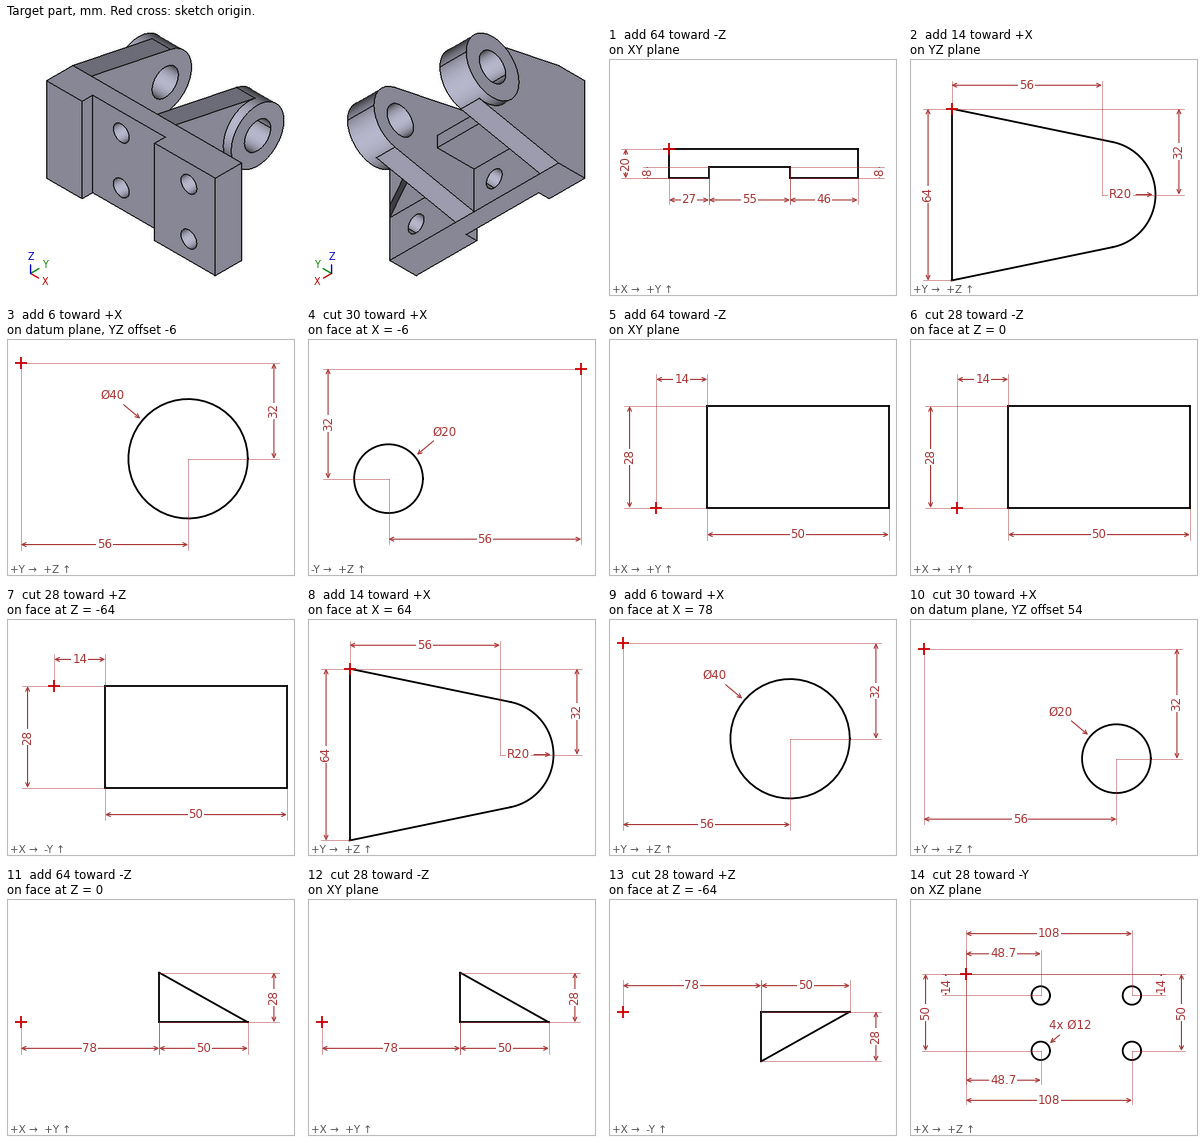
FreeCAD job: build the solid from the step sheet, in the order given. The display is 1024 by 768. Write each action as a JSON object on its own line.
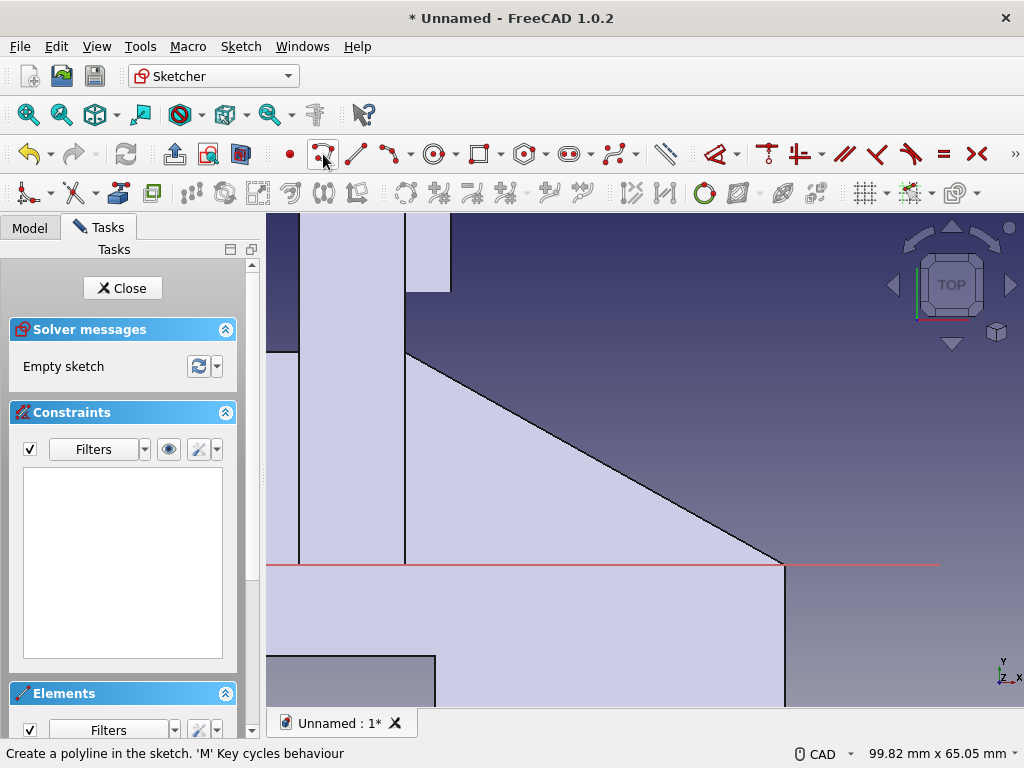
{"action": "left_click", "coordinate": [405, 565]}
{"action": "left_click", "coordinate": [785, 556]}
{"action": "left_click", "coordinate": [405, 352]}
{"action": "left_click", "coordinate": [405, 565]}
{"action": "key", "text": "Escape"}
{"action": "key", "text": "Escape"}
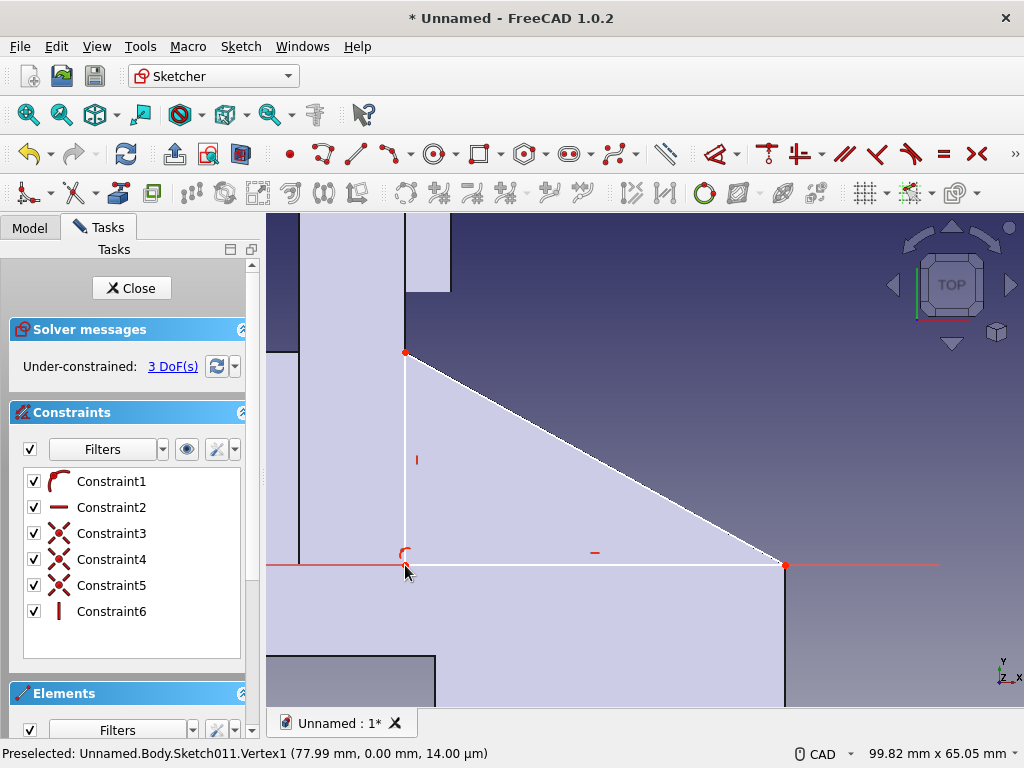
{"action": "left_click", "coordinate": [714, 154]}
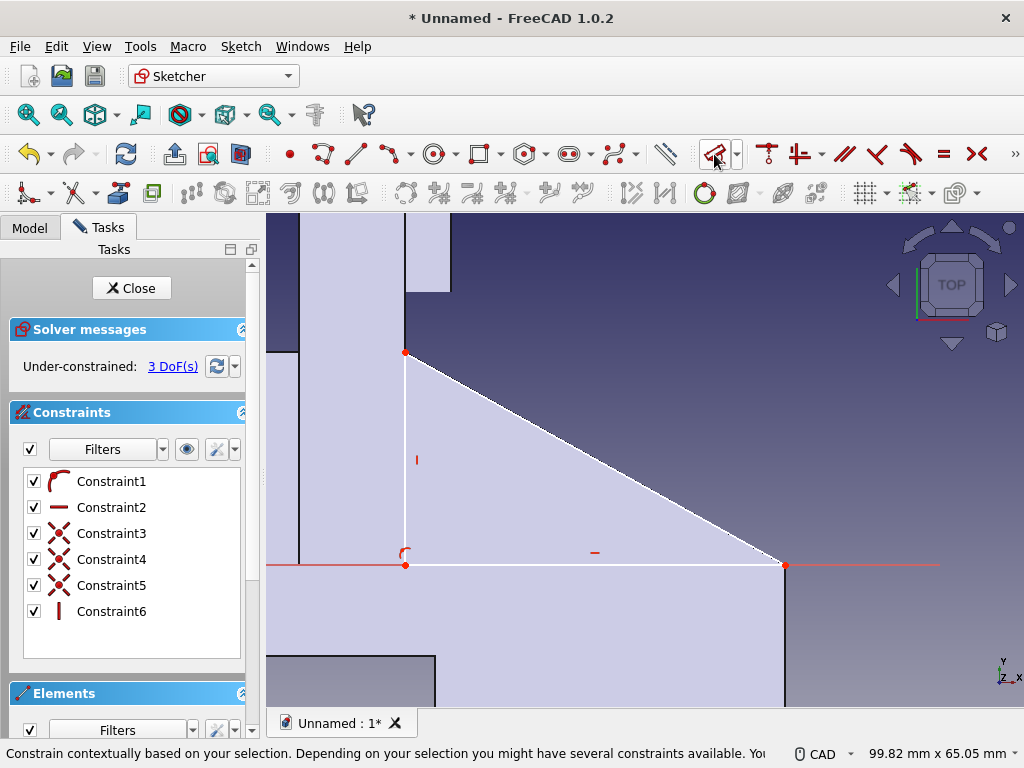
{"action": "left_click", "coordinate": [519, 565]}
{"action": "left_click", "coordinate": [595, 599]}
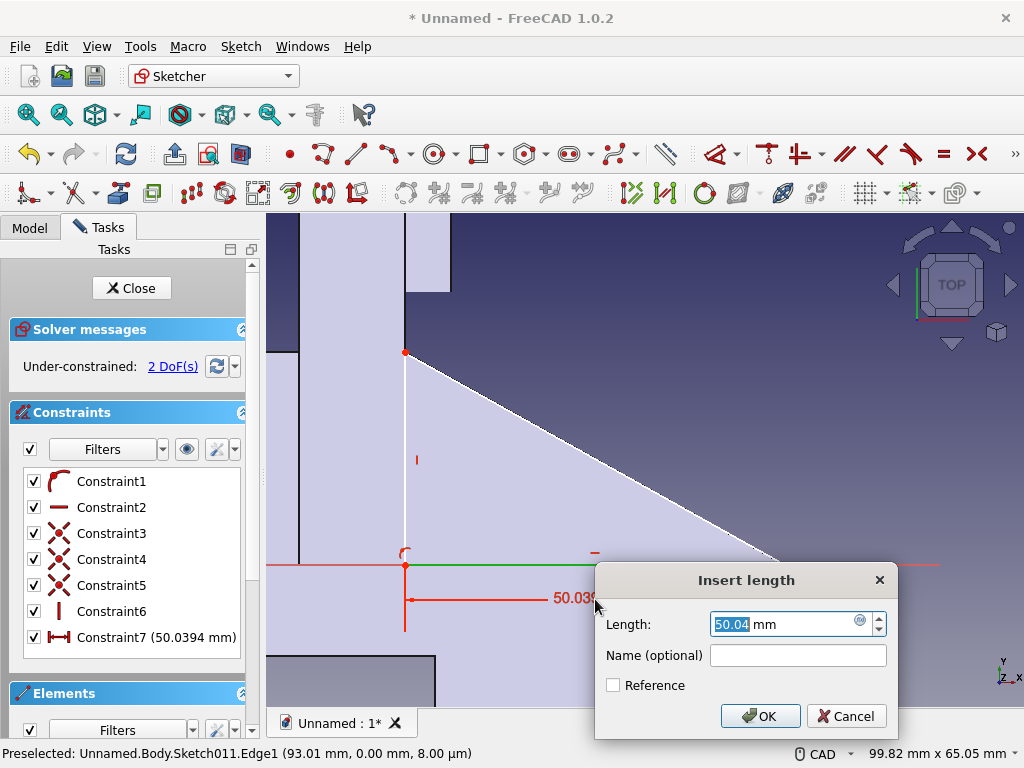
{"action": "type", "text": "50"}
{"action": "key", "text": "Return"}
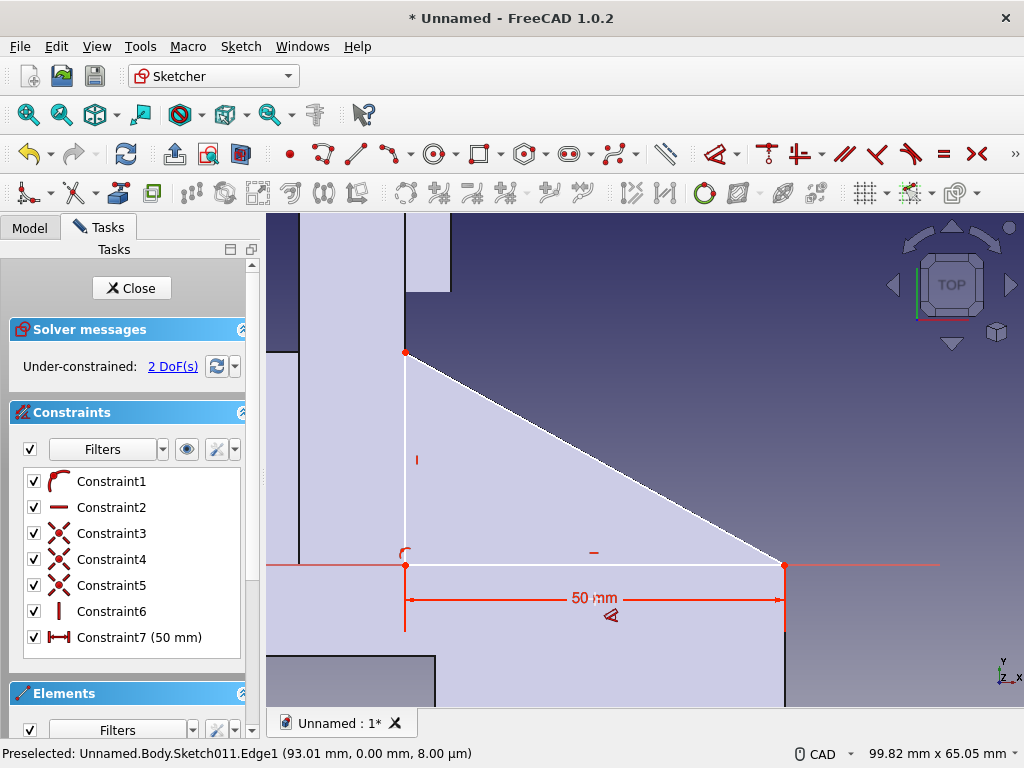
{"action": "left_click", "coordinate": [405, 417]}
{"action": "left_click", "coordinate": [371, 459]}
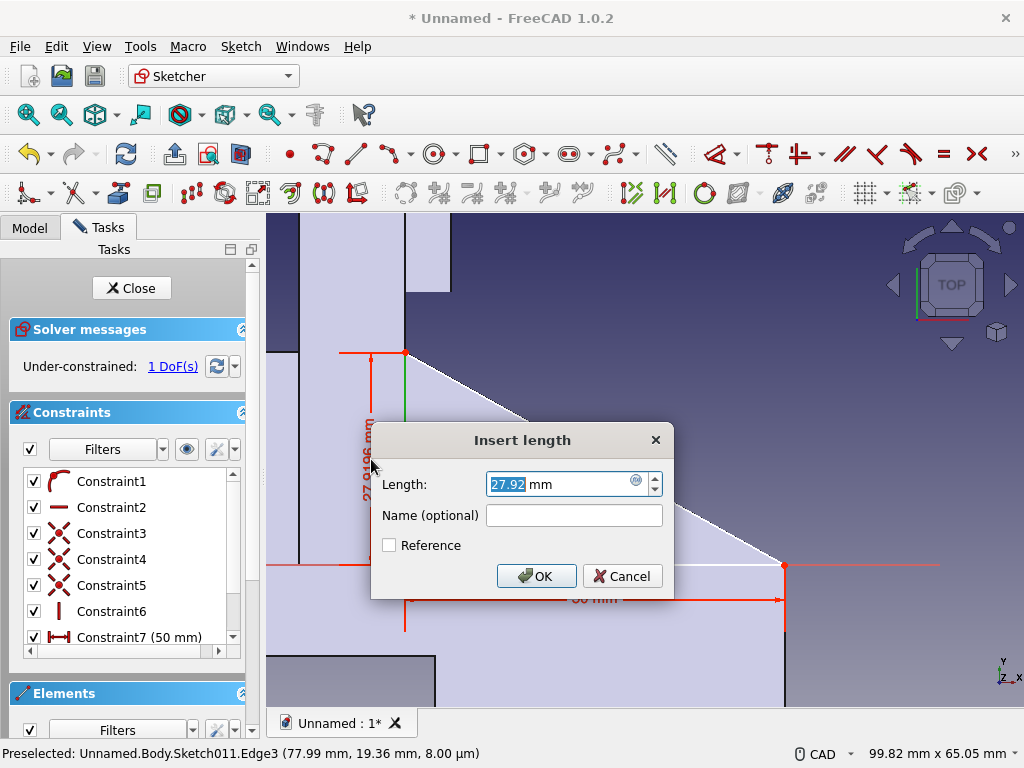
{"action": "type", "text": "28"}
{"action": "key", "text": "Return"}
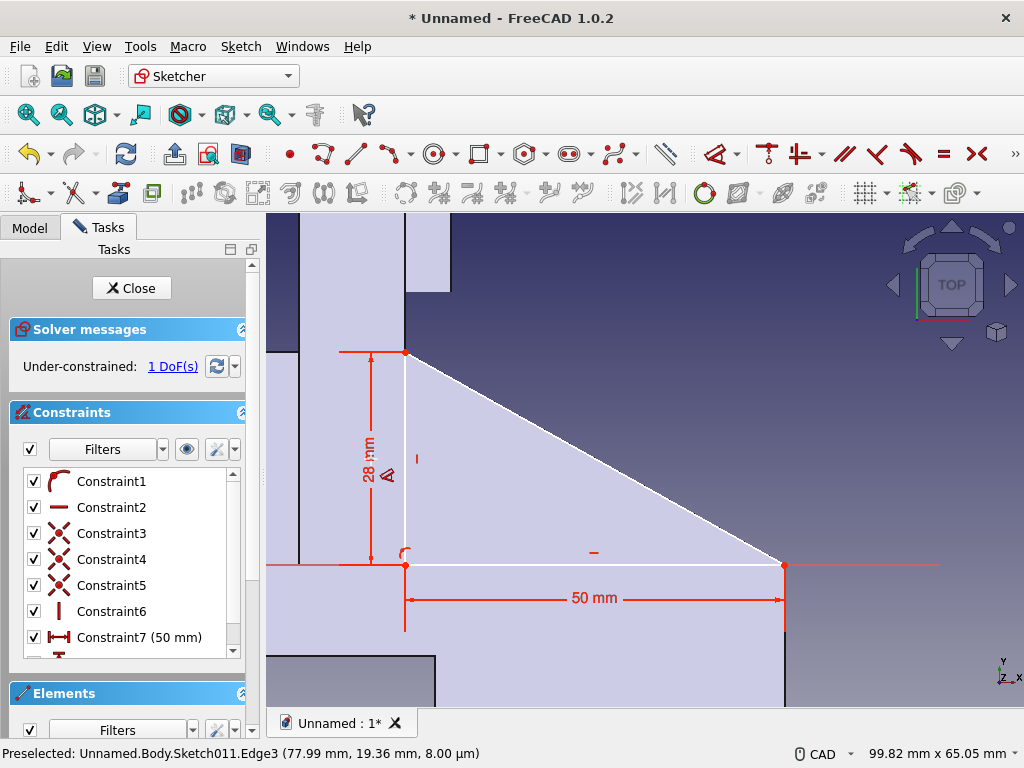
{"action": "left_click", "coordinate": [405, 565]}
{"action": "left_click", "coordinate": [350, 599]}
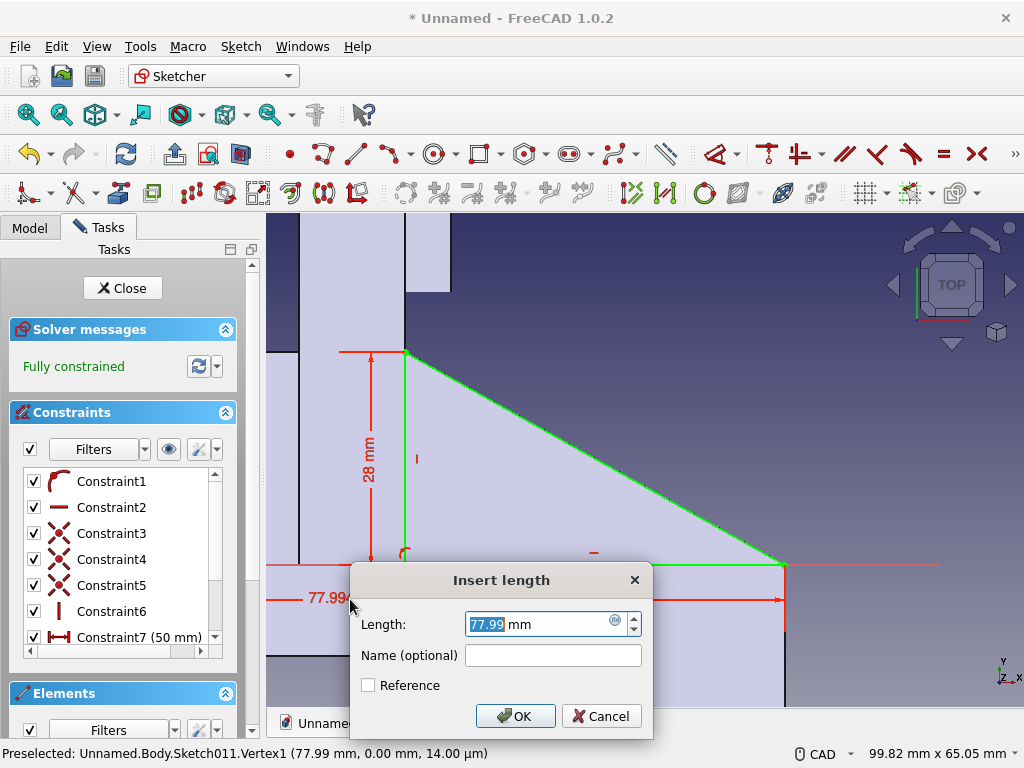
{"action": "type", "text": "78"}
{"action": "key", "text": "Return"}
{"action": "key", "text": "Escape"}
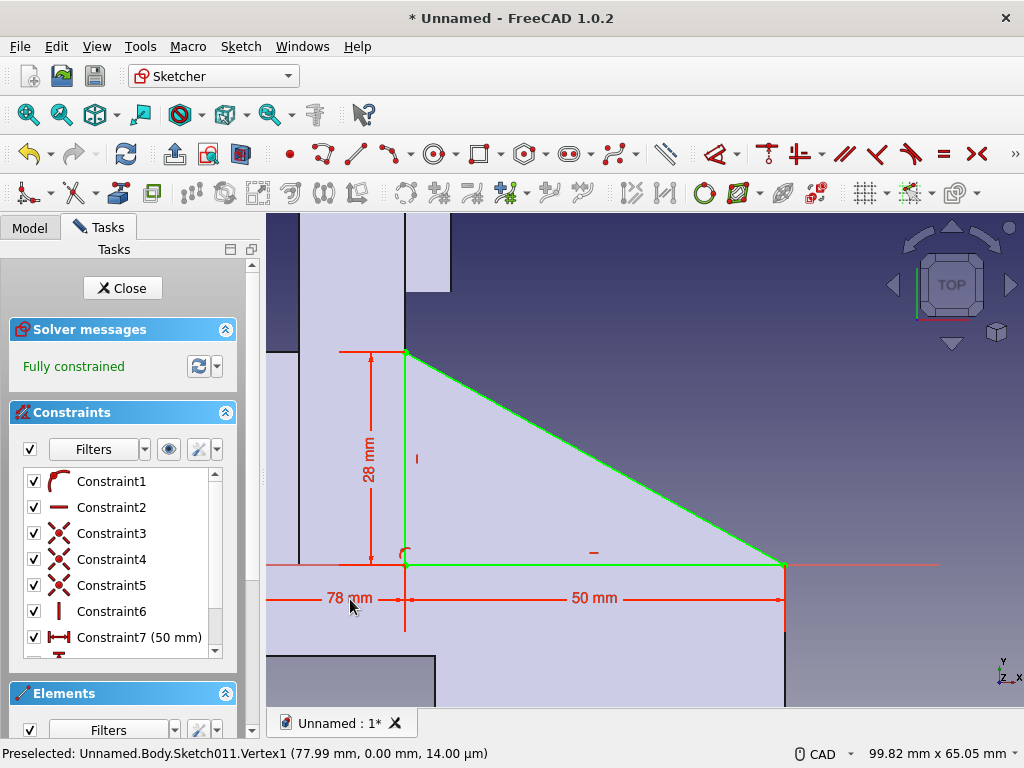
{"action": "left_click", "coordinate": [123, 288]}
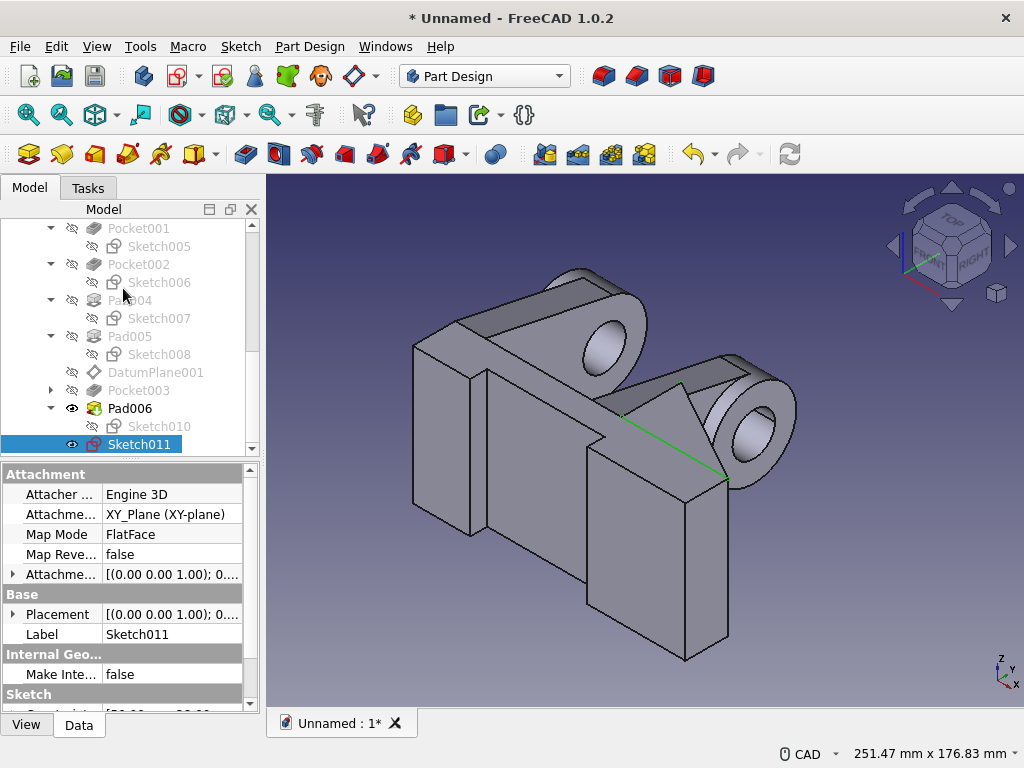
{"action": "left_click", "coordinate": [246, 154]}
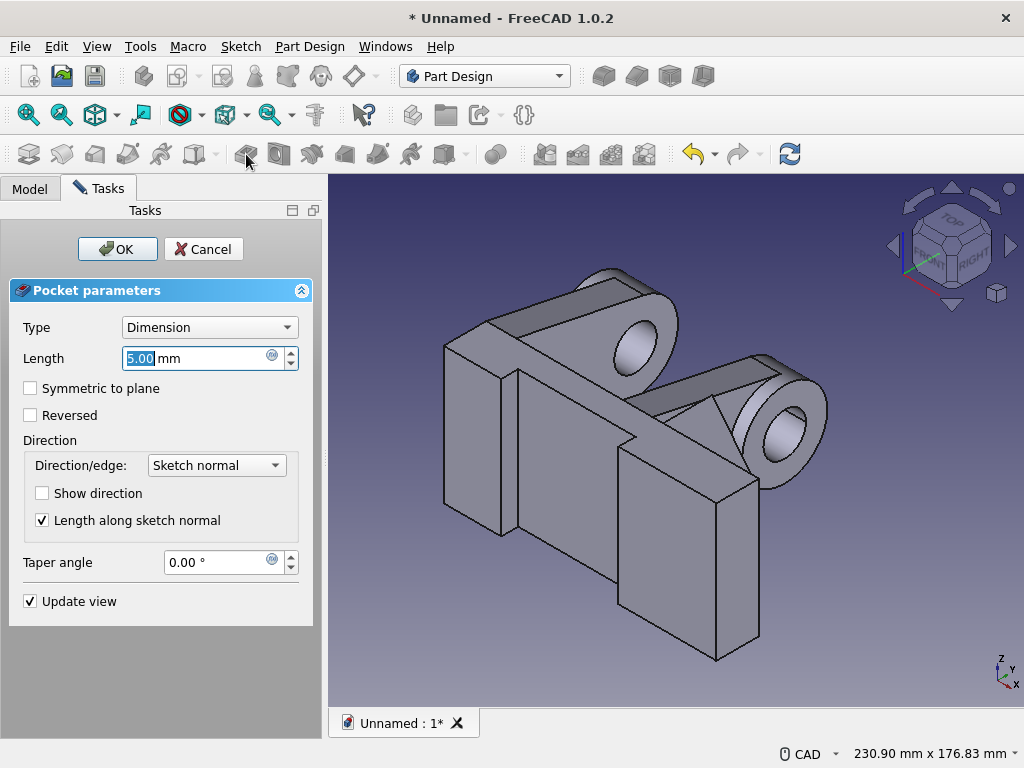
{"action": "type", "text": "28"}
{"action": "key", "text": "Tab"}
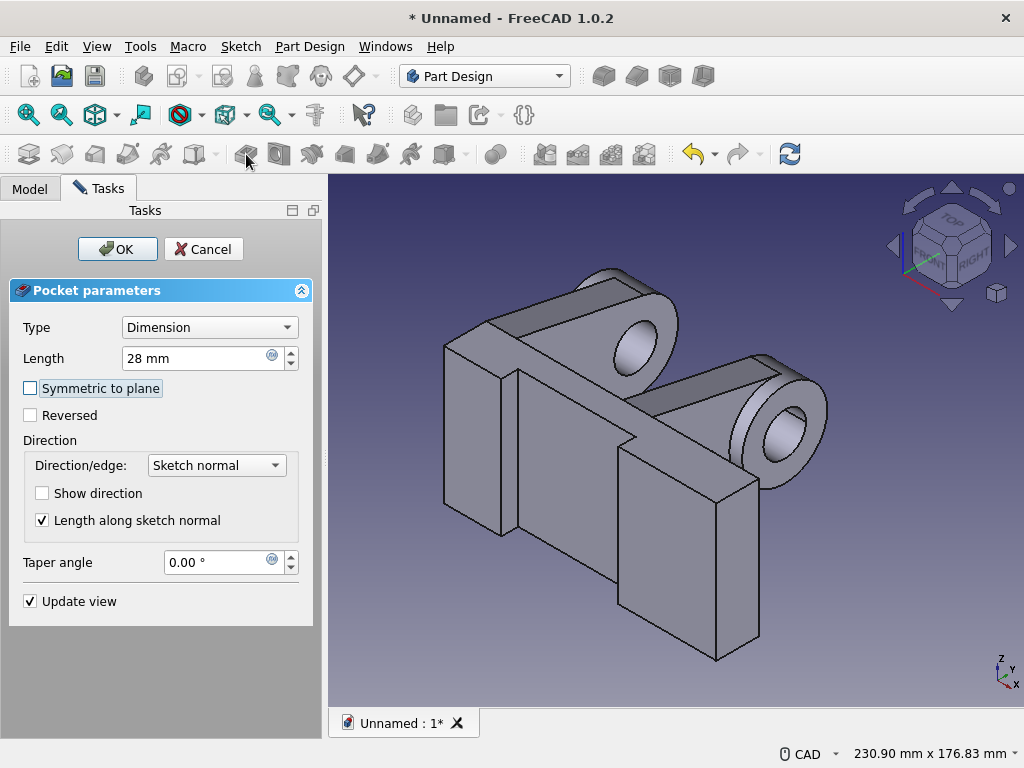
{"action": "left_click", "coordinate": [118, 249]}